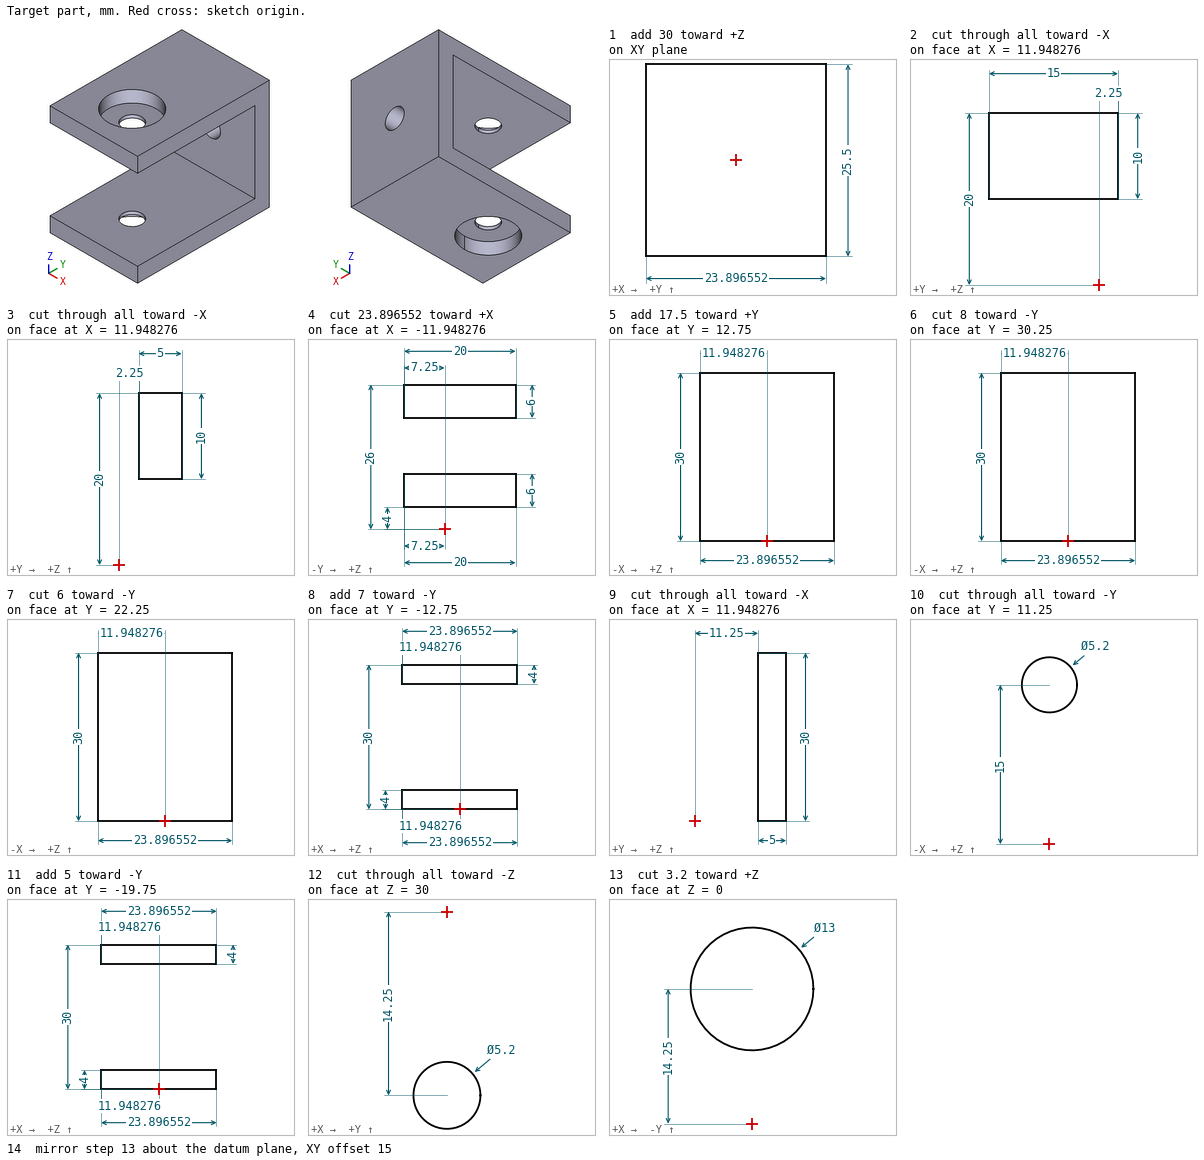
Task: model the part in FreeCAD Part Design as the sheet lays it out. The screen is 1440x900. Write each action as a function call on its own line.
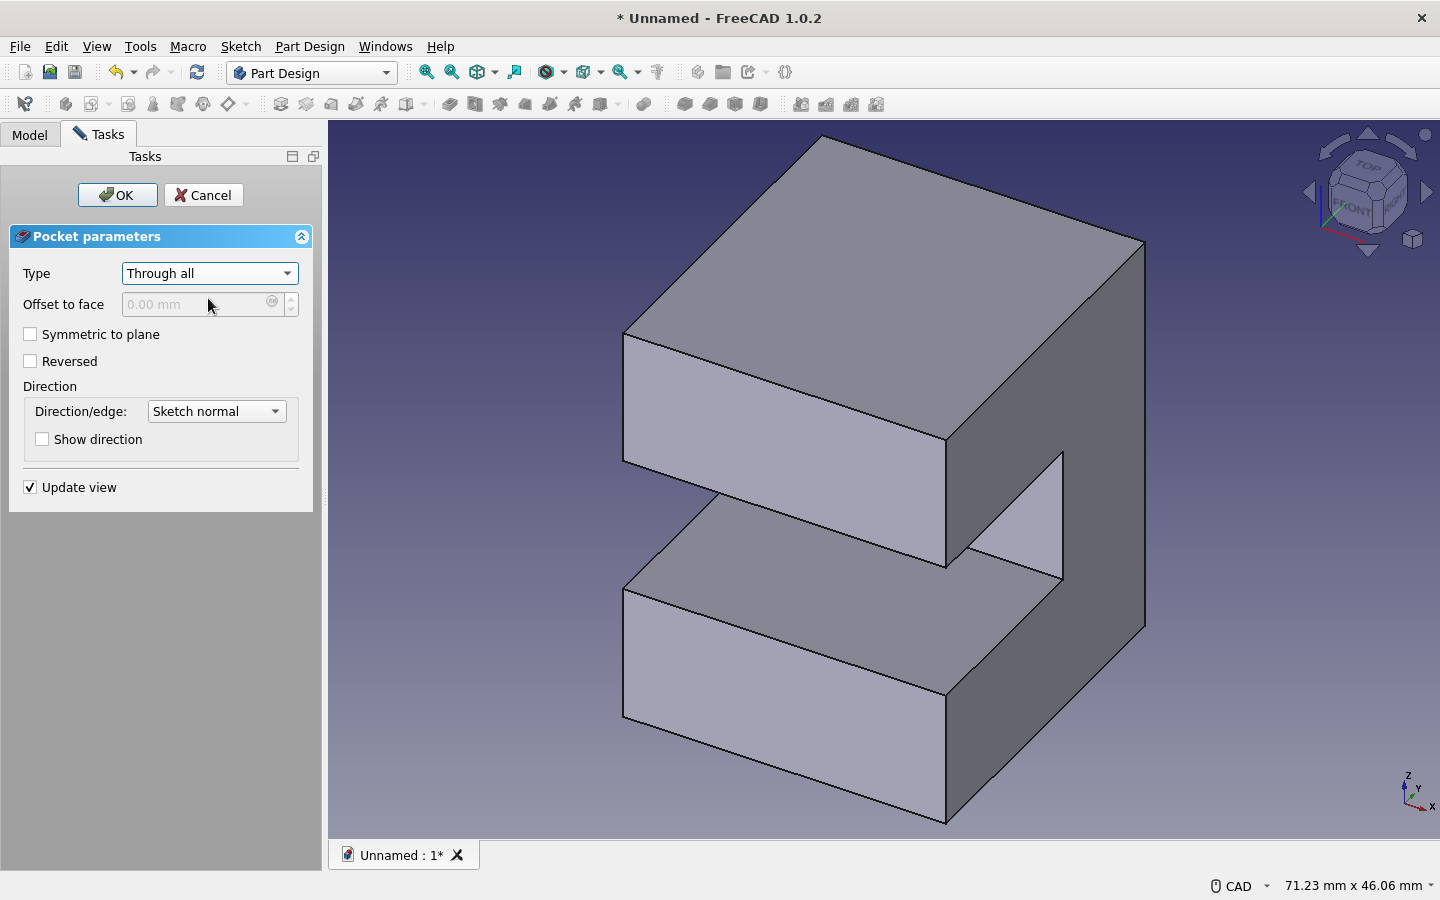
click(118, 195)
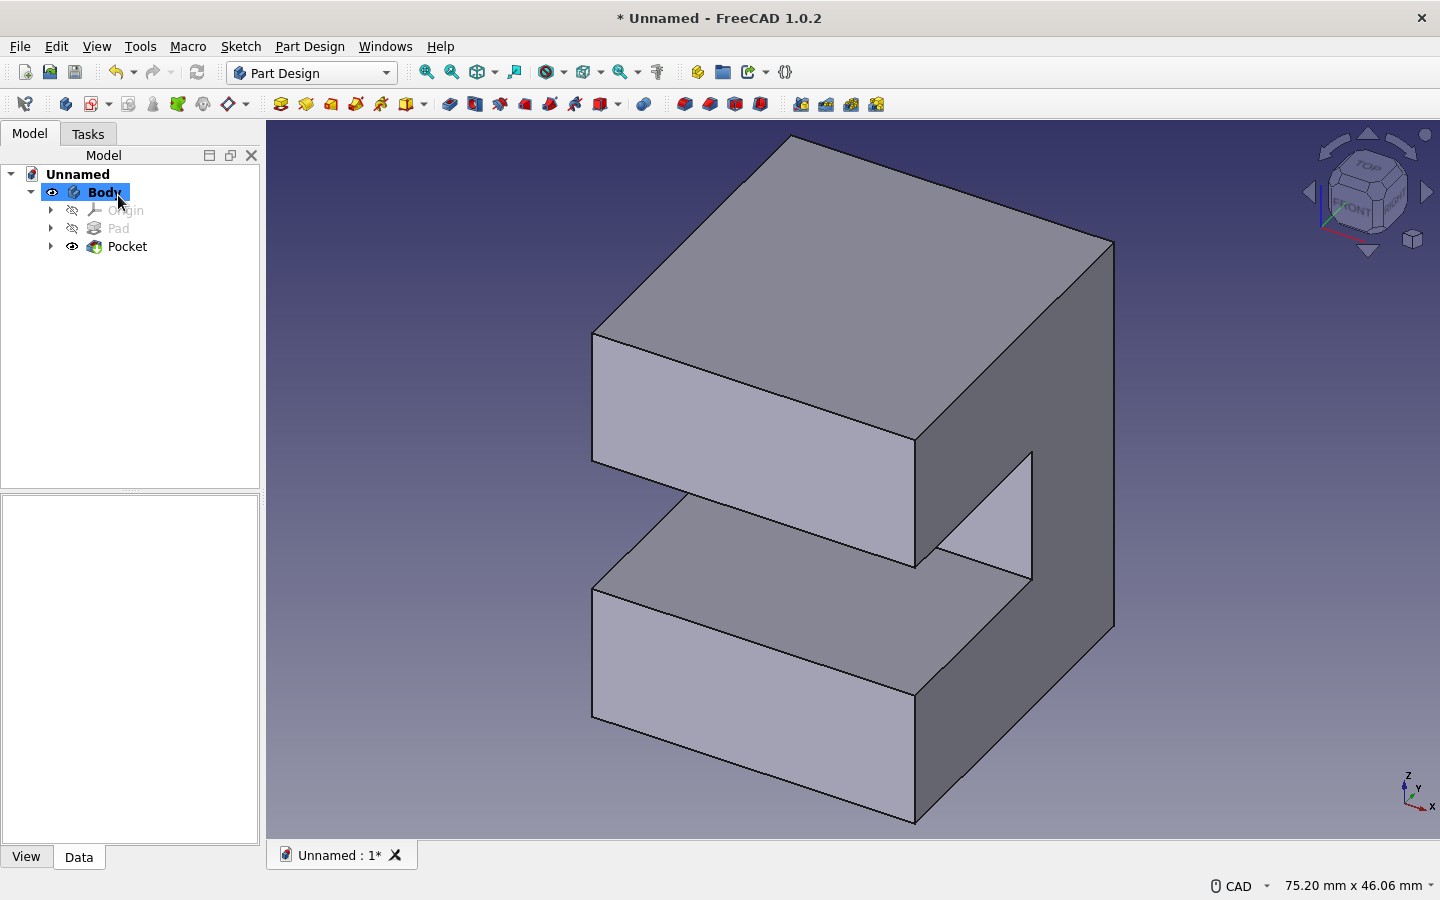
click(1071, 366)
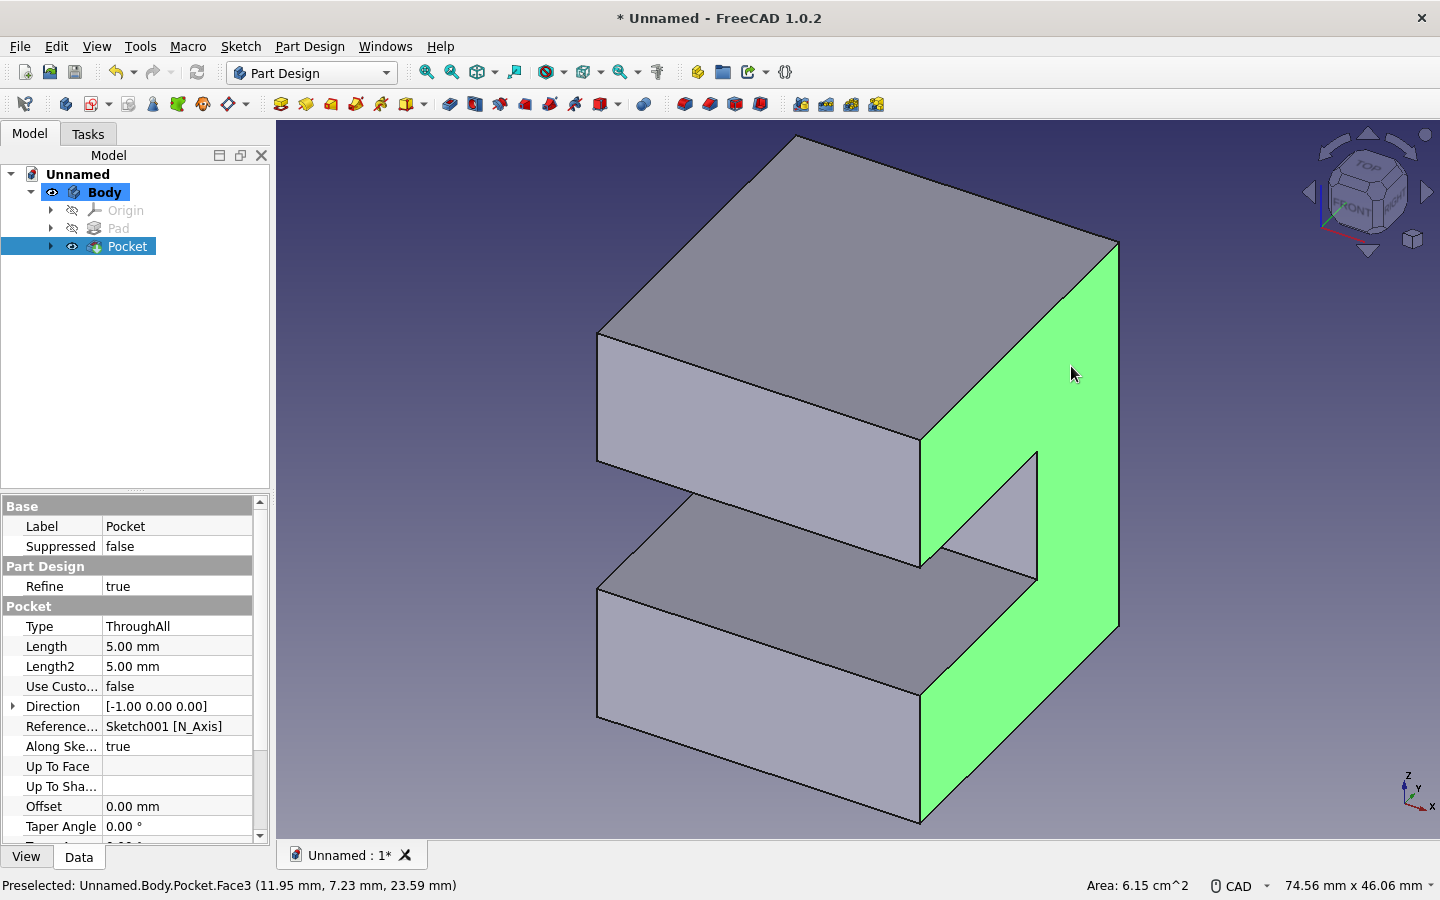
click(90, 104)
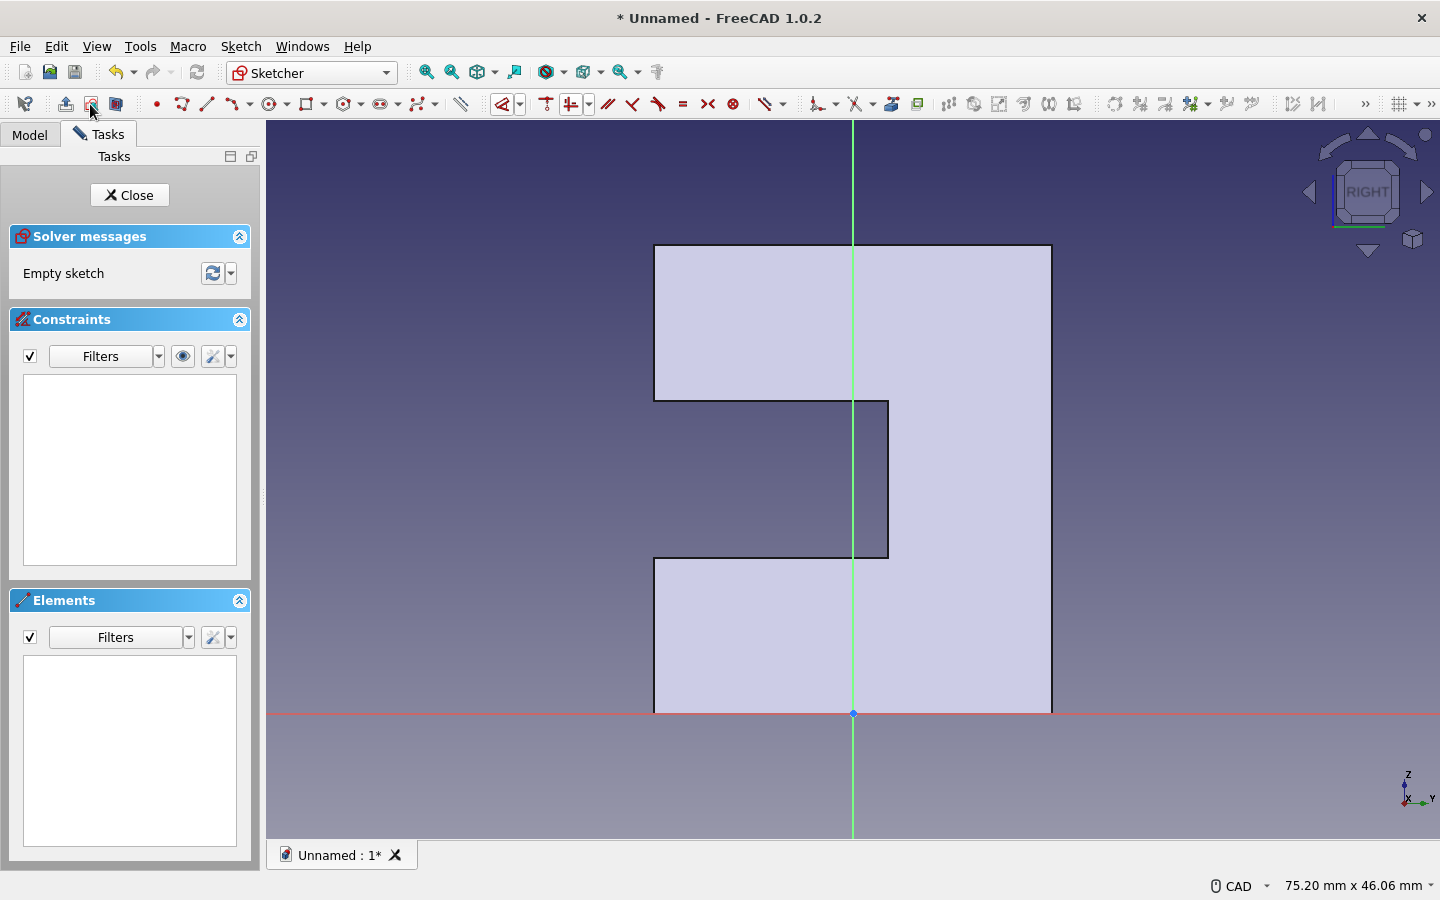
scroll(1164, 716, up, 2)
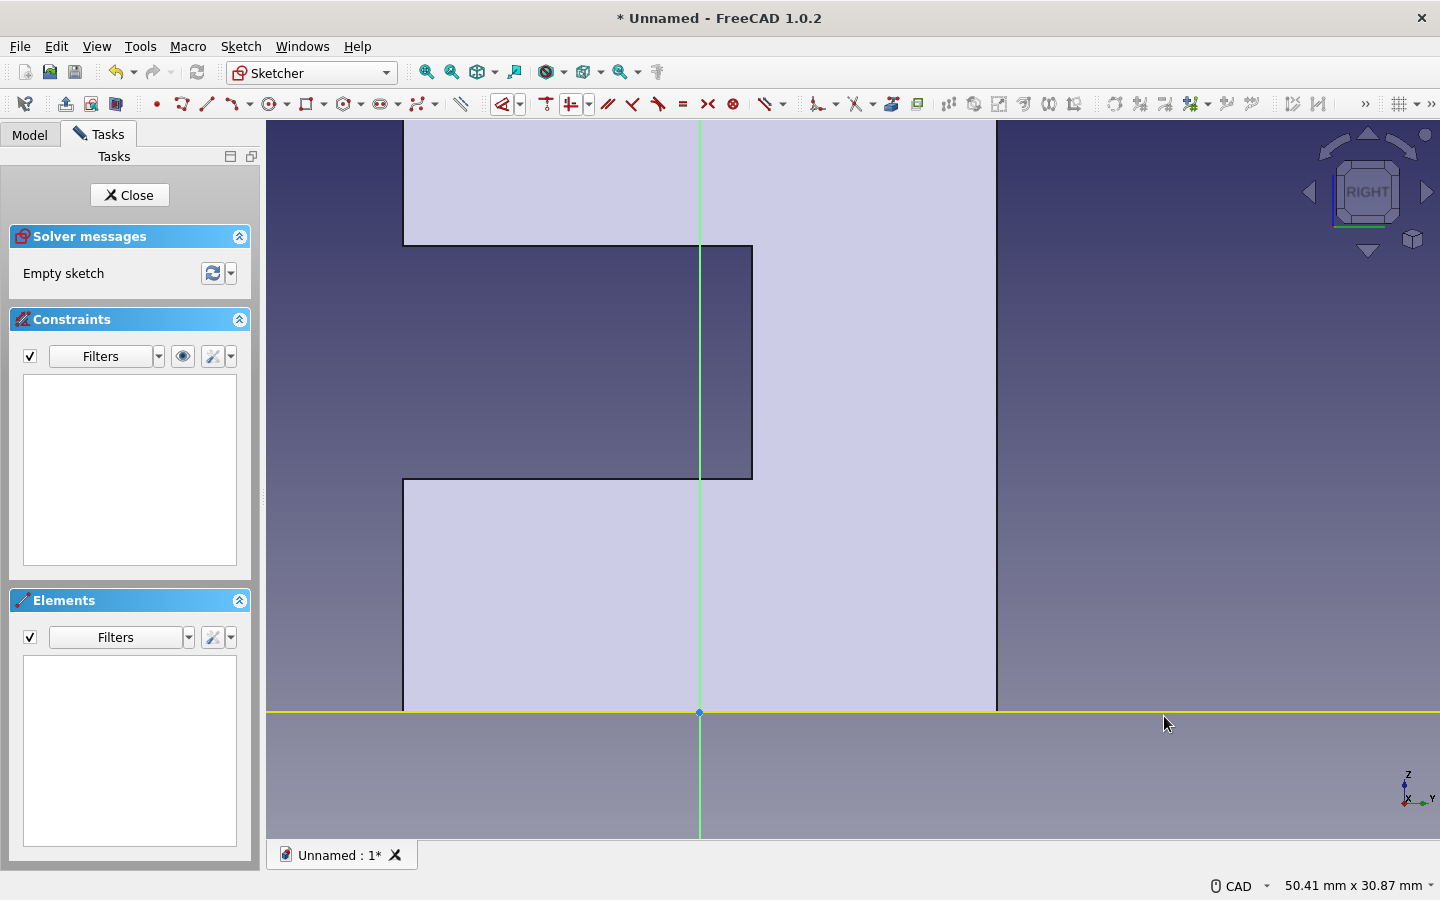
key(g)
key(r)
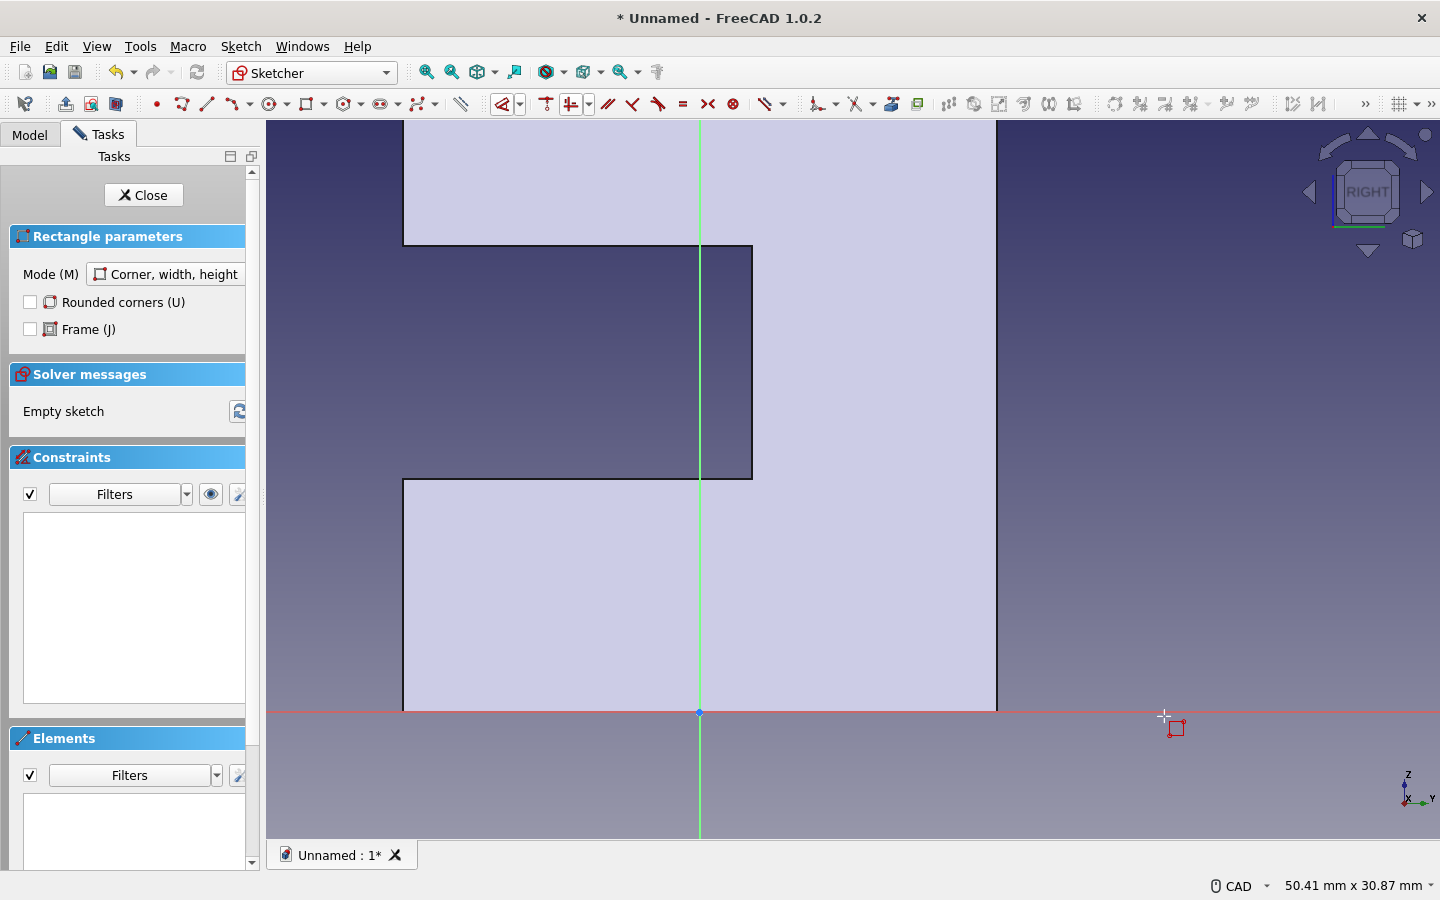
click(752, 246)
move(869, 479)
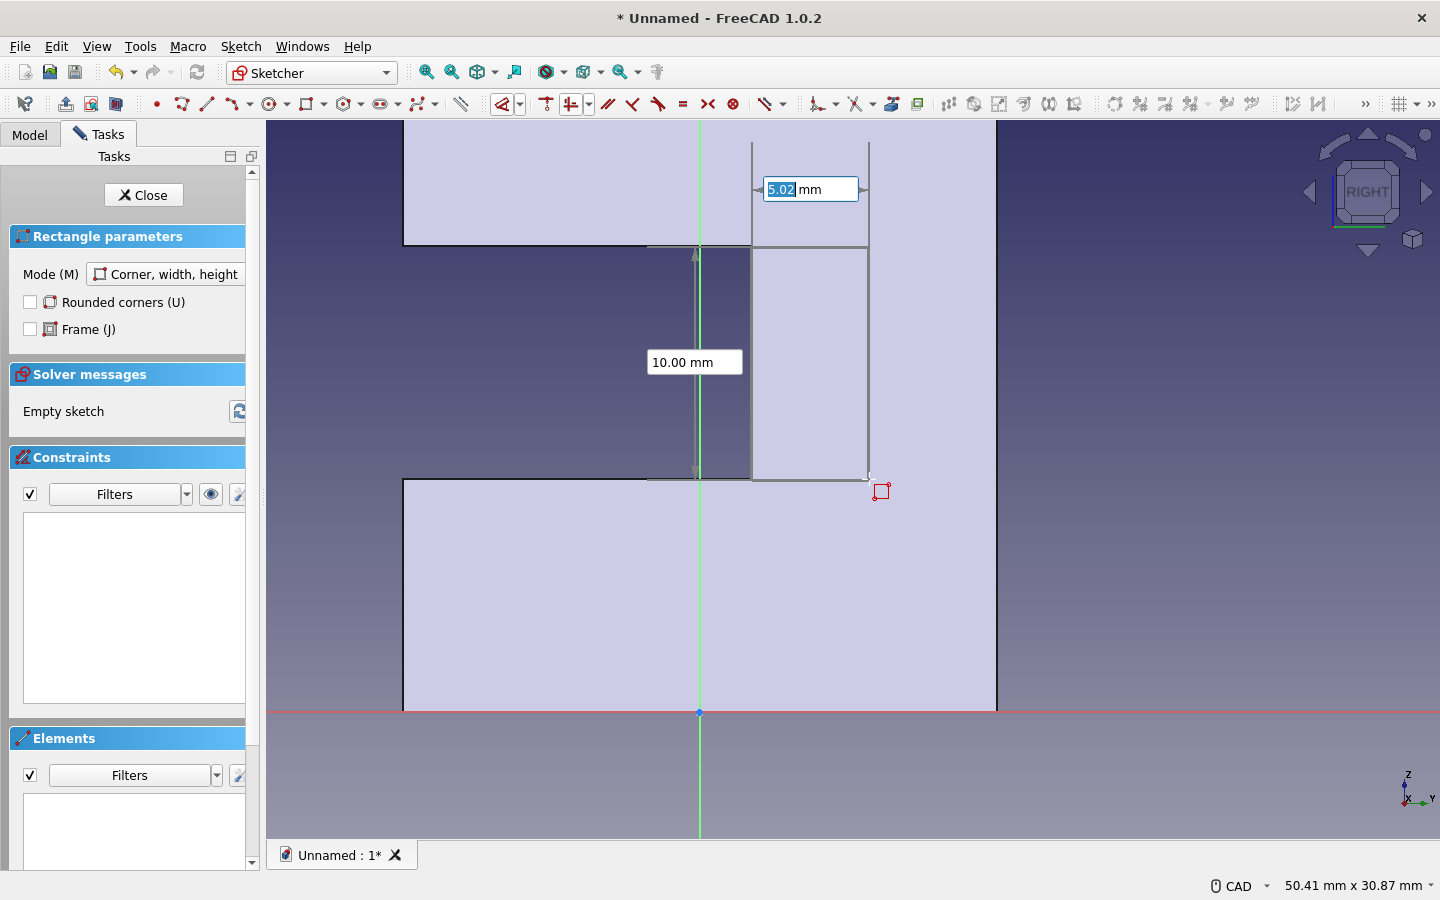
text(5)
key(Tab)
text(10)
key(Return)
key(Escape)